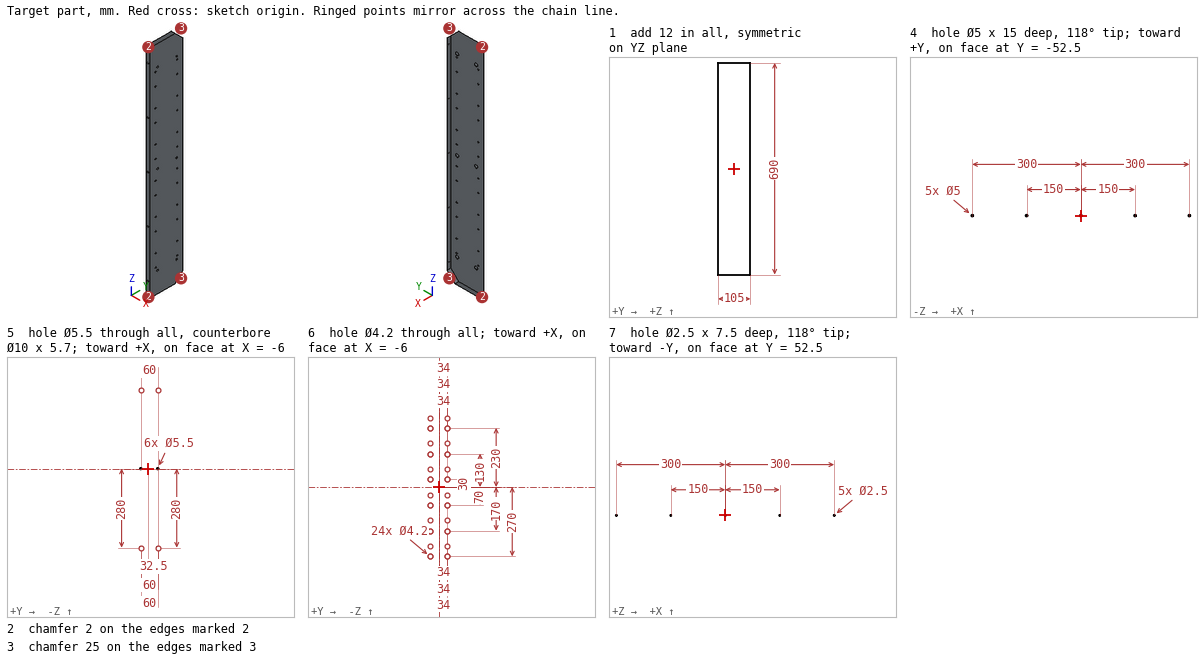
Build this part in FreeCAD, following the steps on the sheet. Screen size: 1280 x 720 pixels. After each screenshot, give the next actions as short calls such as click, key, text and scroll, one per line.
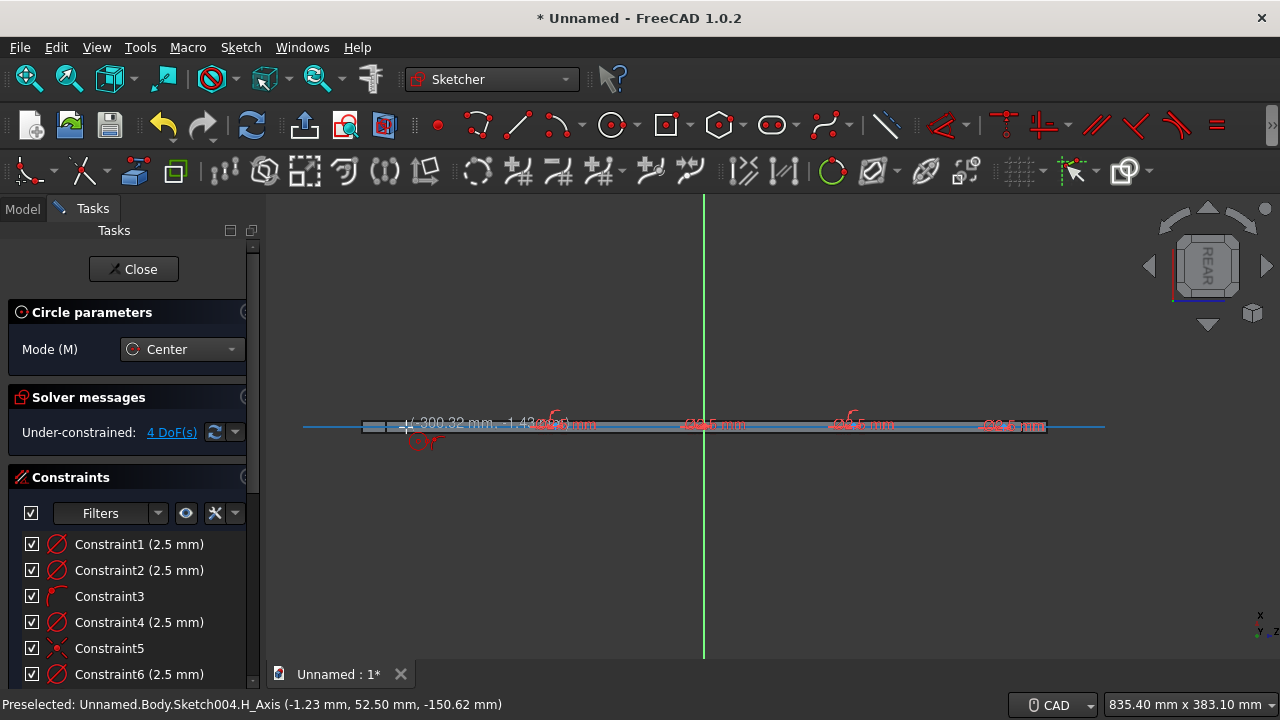
click(406, 427)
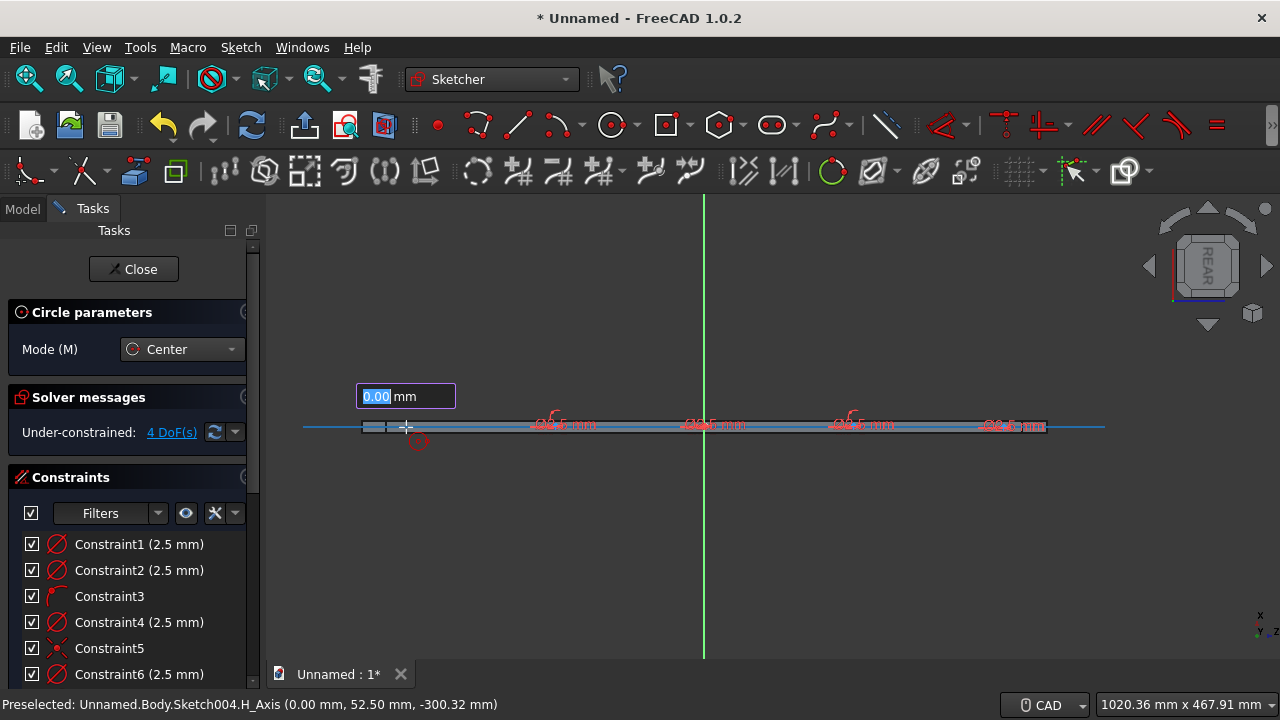
scroll(406, 428, up, 14)
move(402, 416)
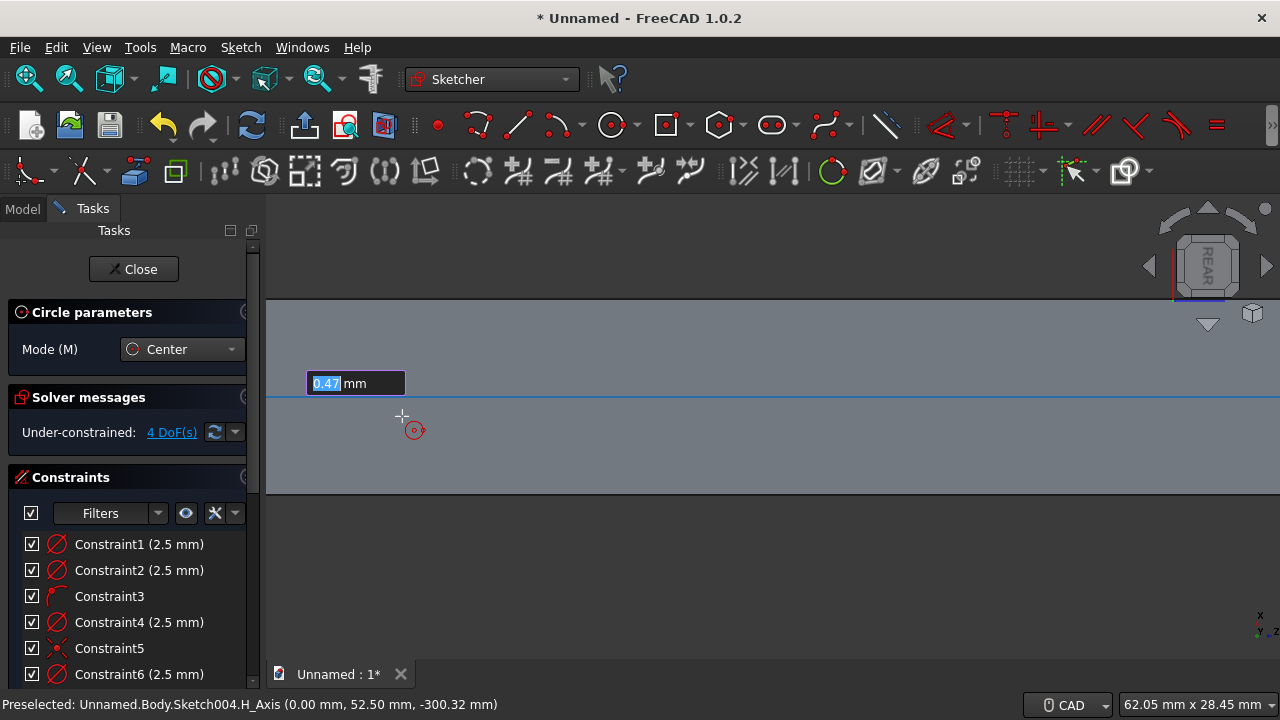
text(2.5)
key(Return)
key(Escape)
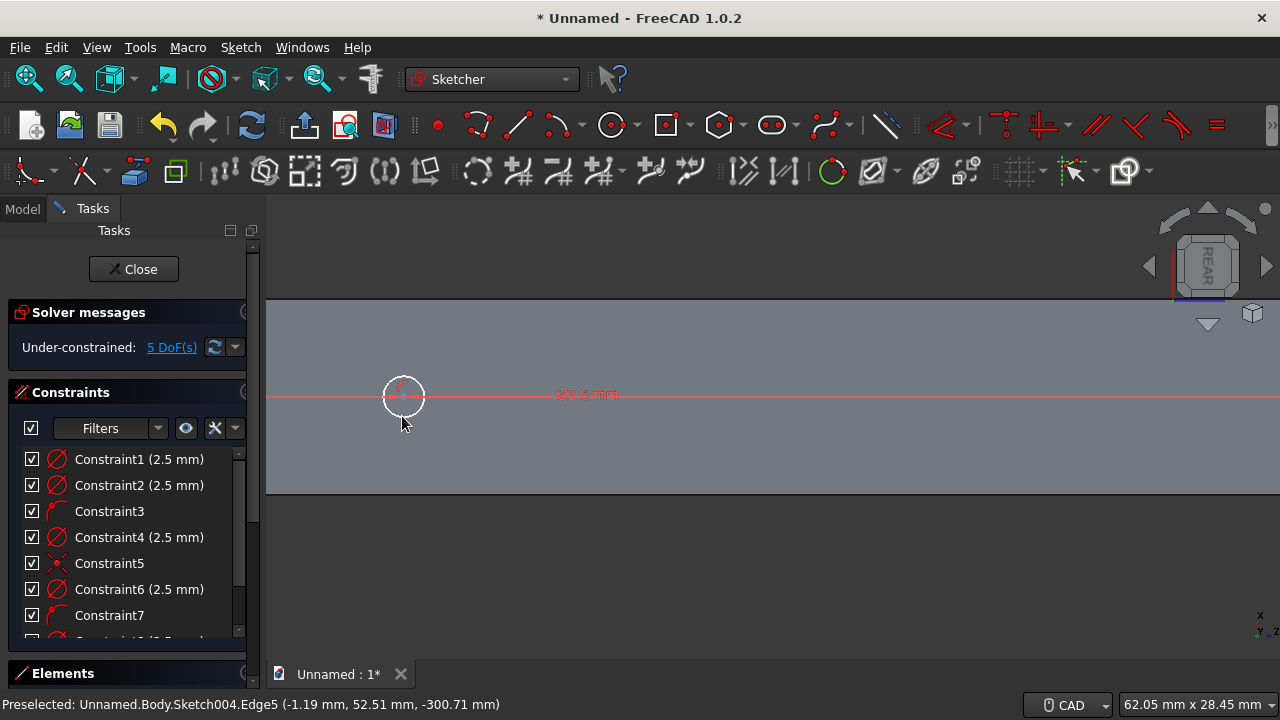
scroll(406, 428, down, 14)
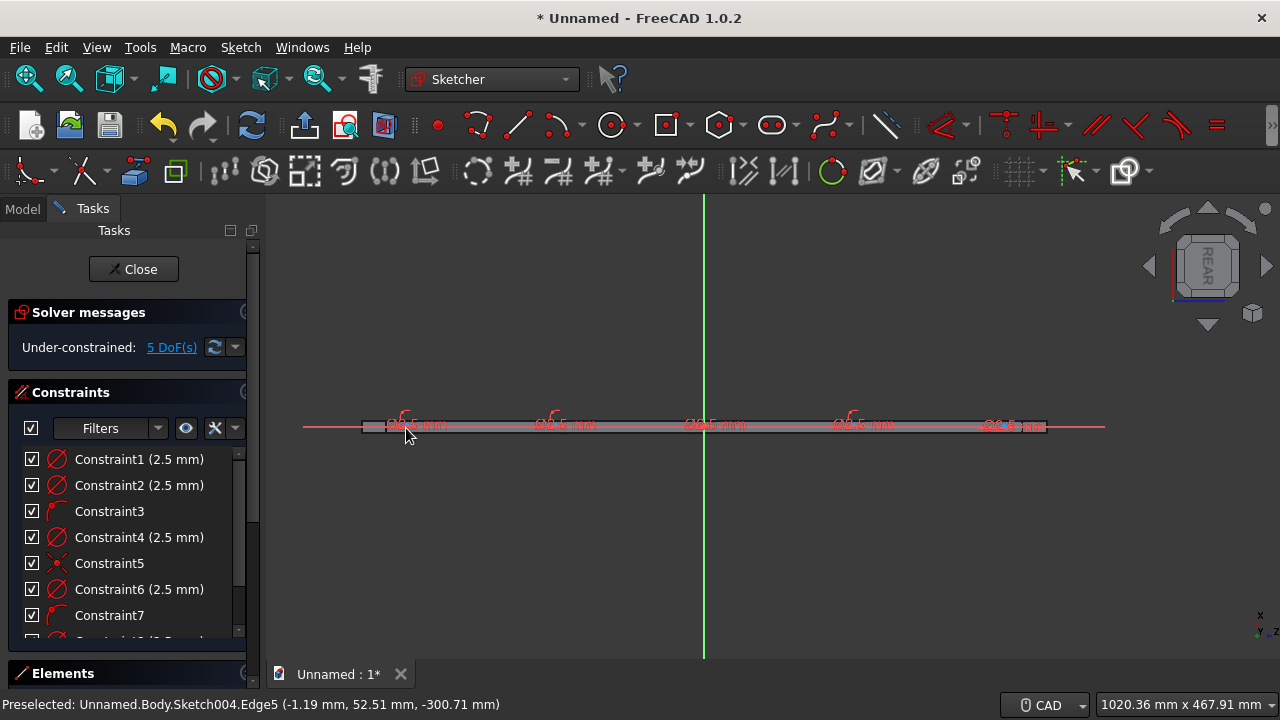
click(1003, 428)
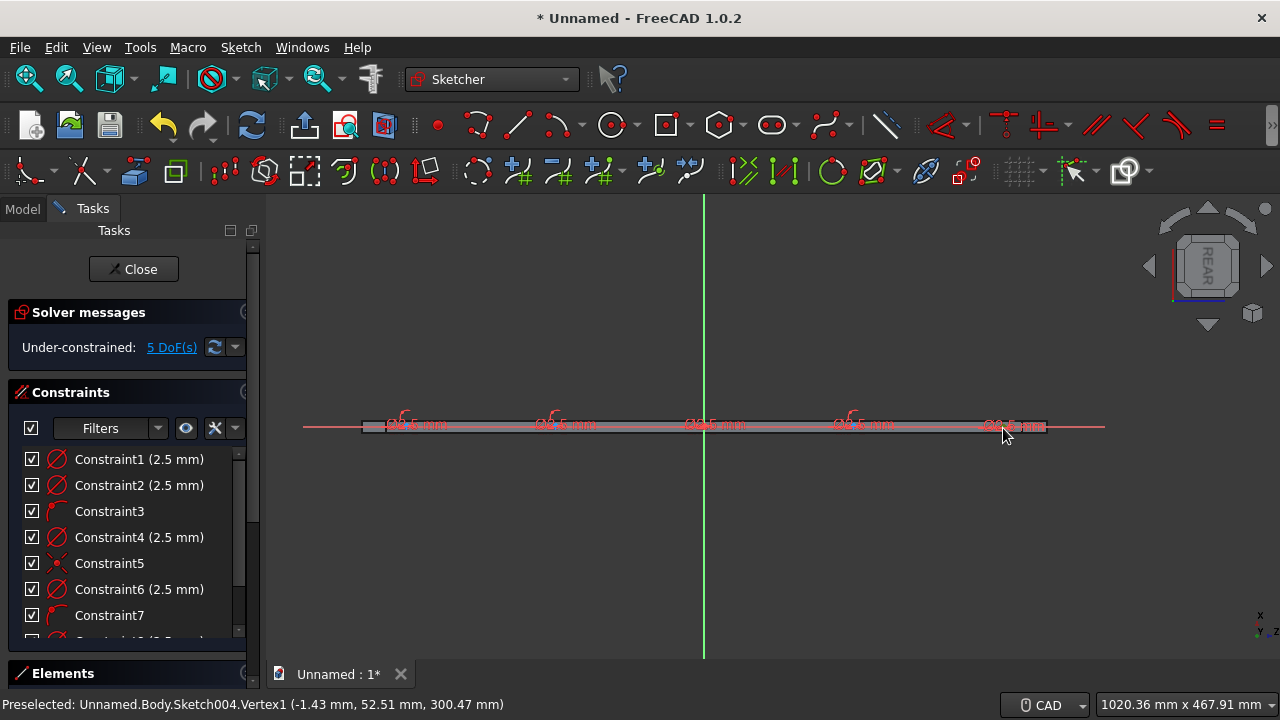
click(353, 427)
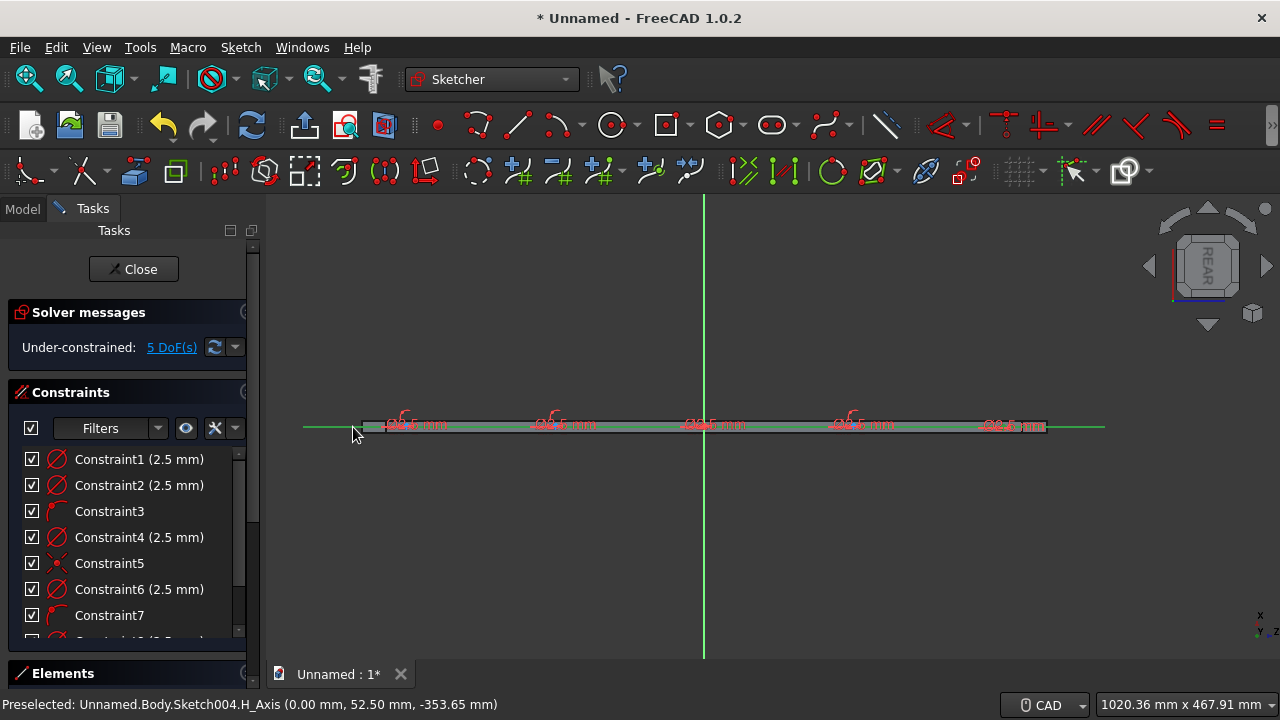
click(1004, 126)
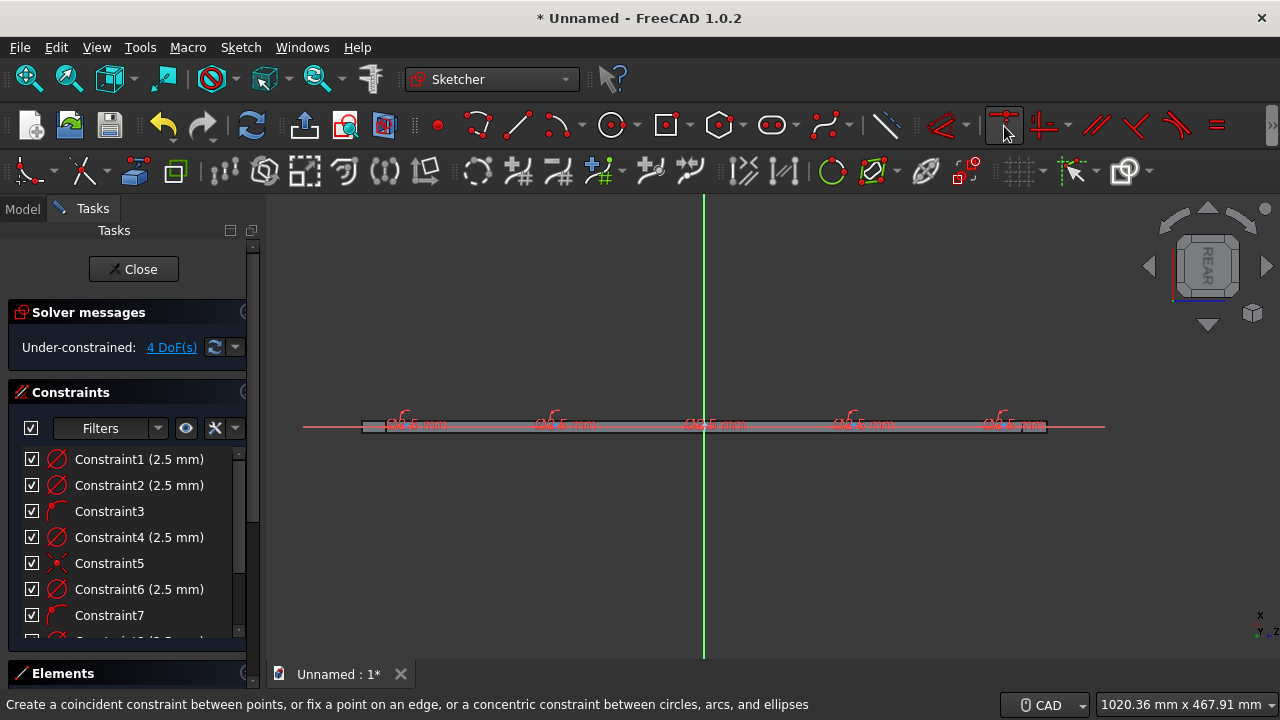
click(942, 126)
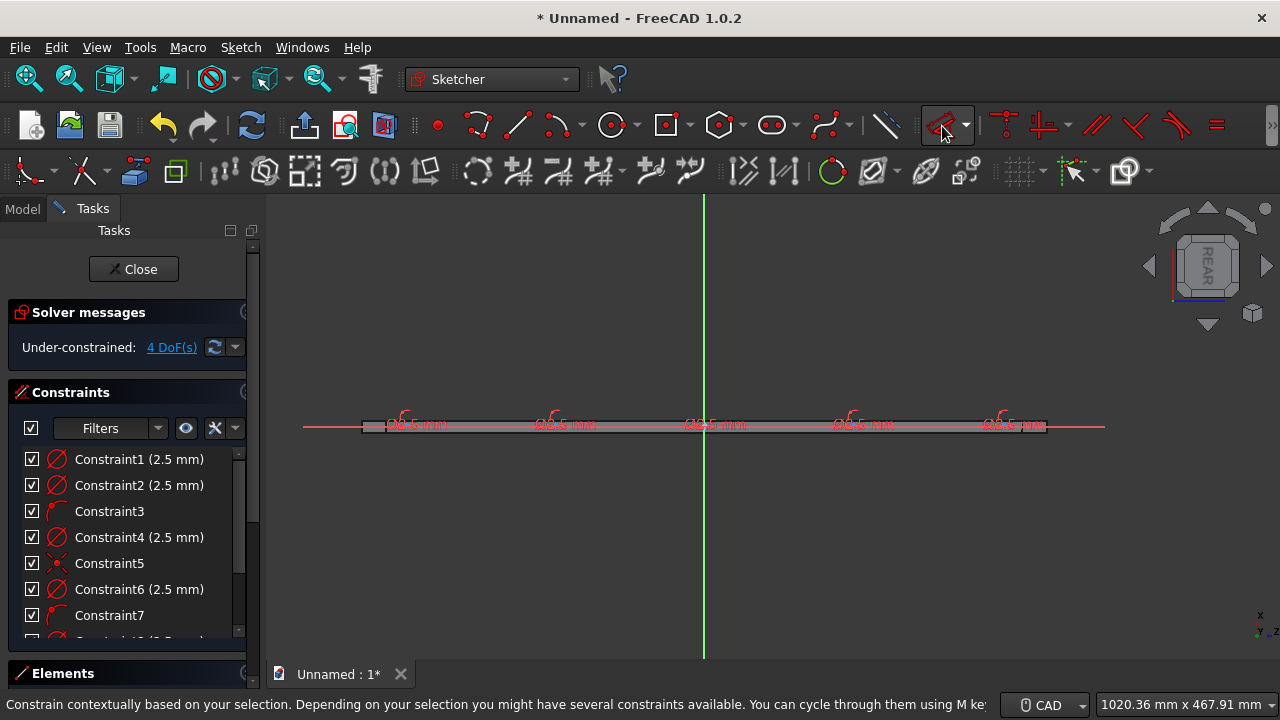
click(1003, 427)
click(854, 461)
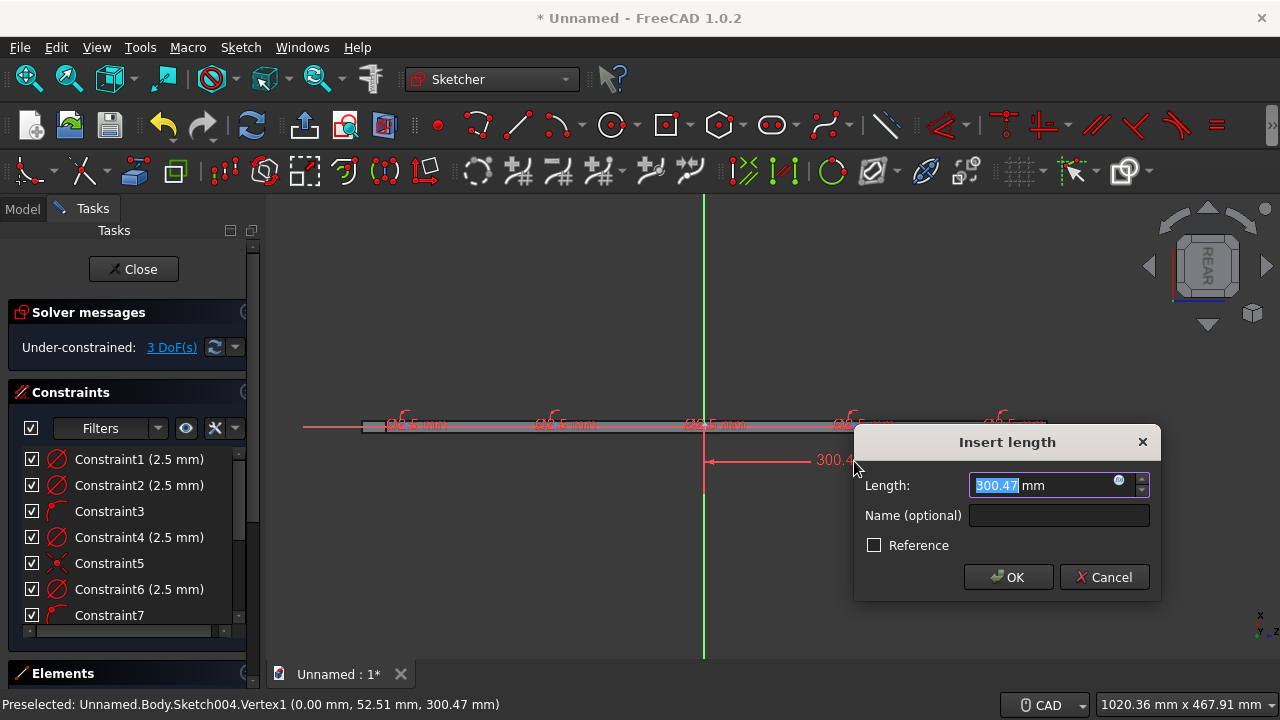
text(300)
key(Return)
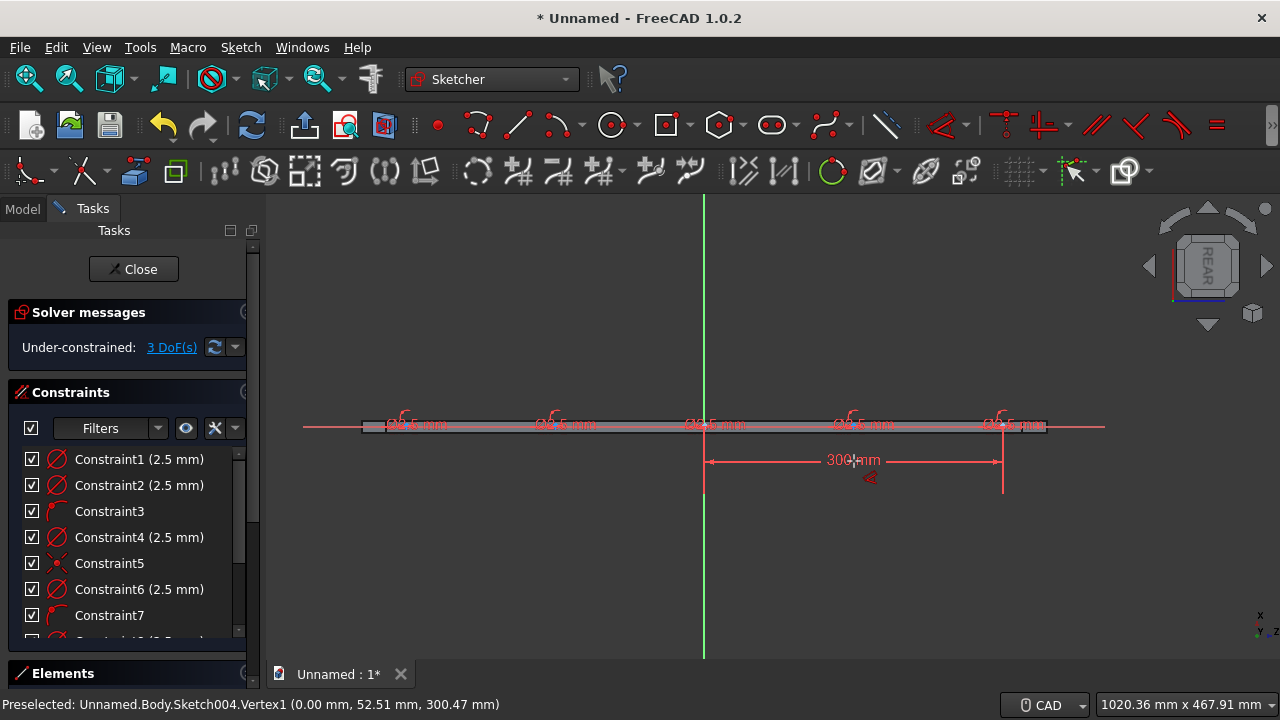
click(853, 427)
click(779, 461)